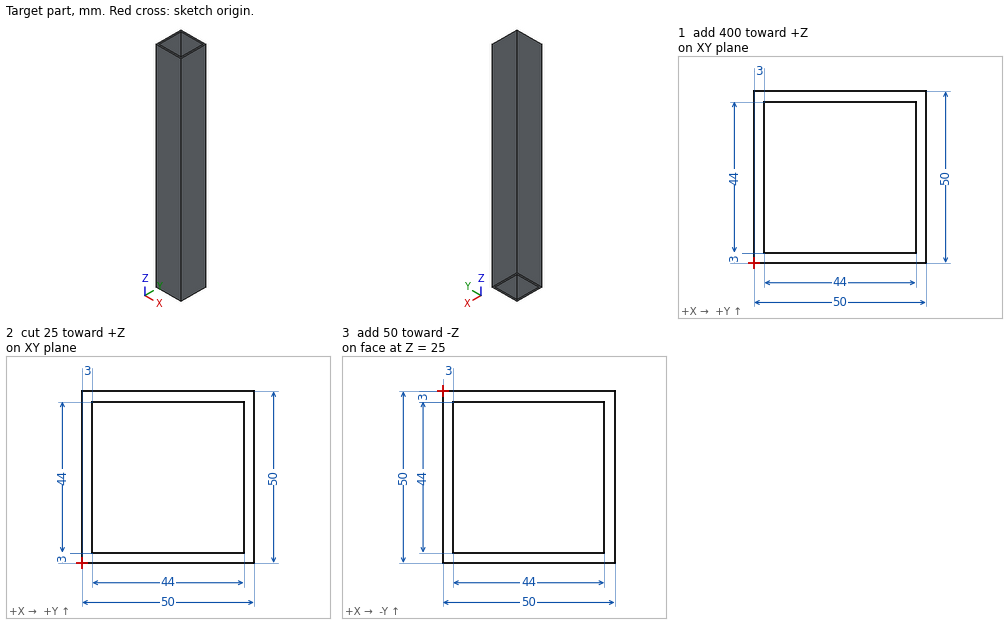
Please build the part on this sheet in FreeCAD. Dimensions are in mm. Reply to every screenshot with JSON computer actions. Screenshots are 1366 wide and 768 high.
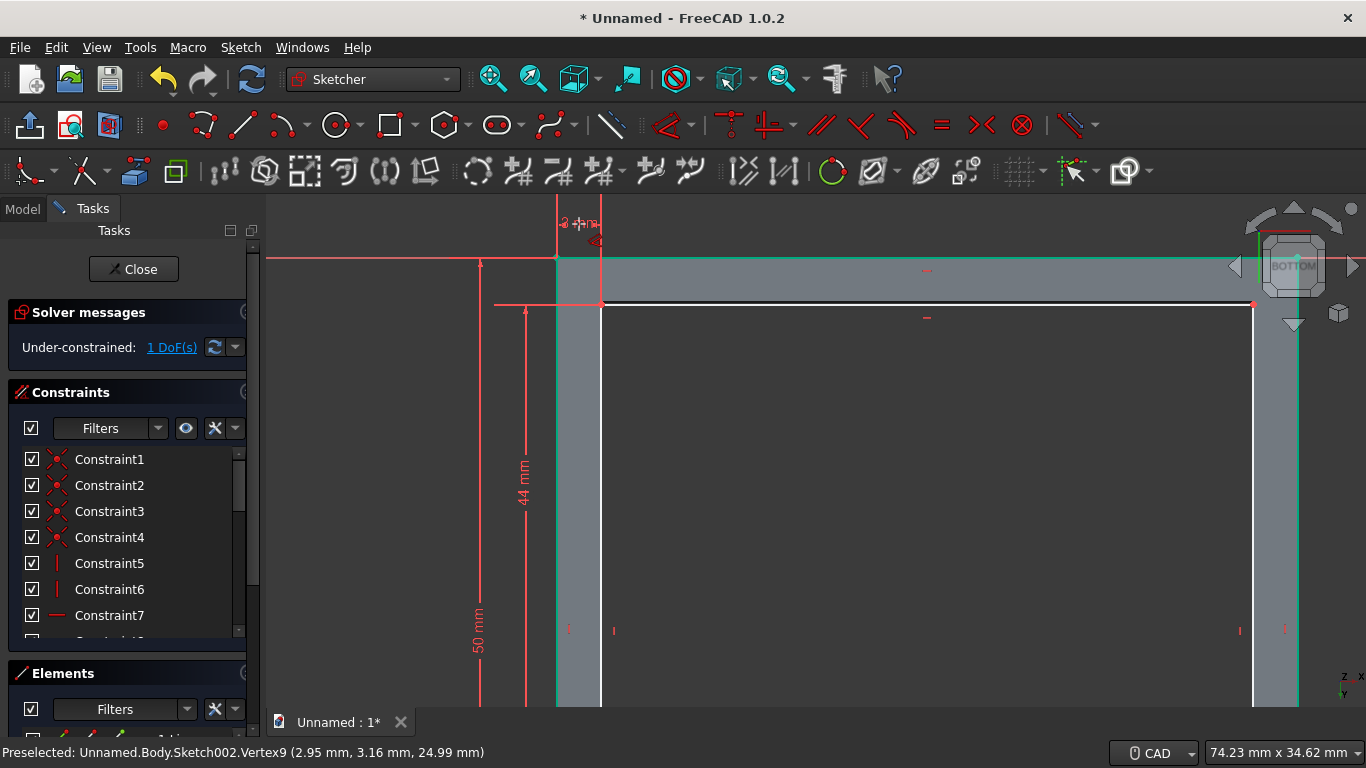
{"action": "left_click", "coordinate": [601, 305]}
{"action": "left_click", "coordinate": [523, 281]}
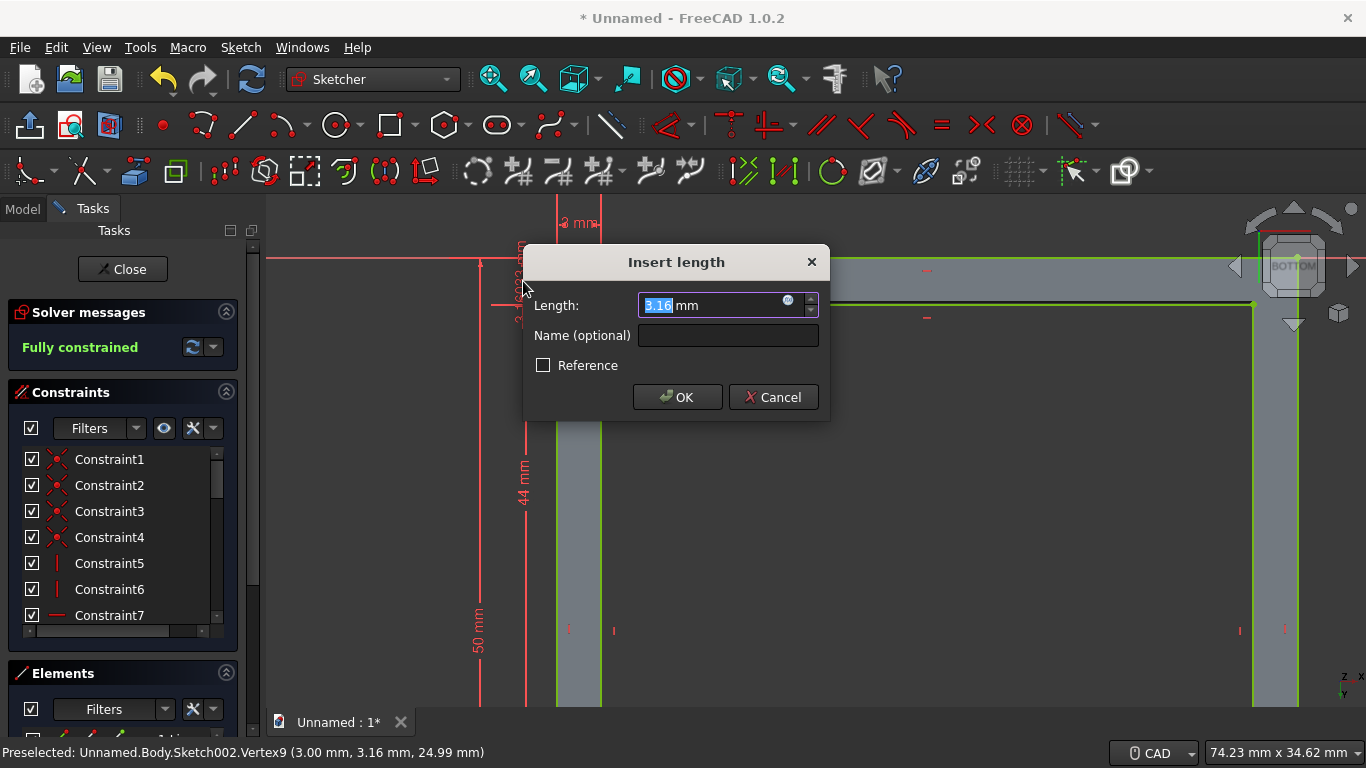
{"action": "type", "text": "3"}
{"action": "key", "text": "Return"}
{"action": "key", "text": "Escape"}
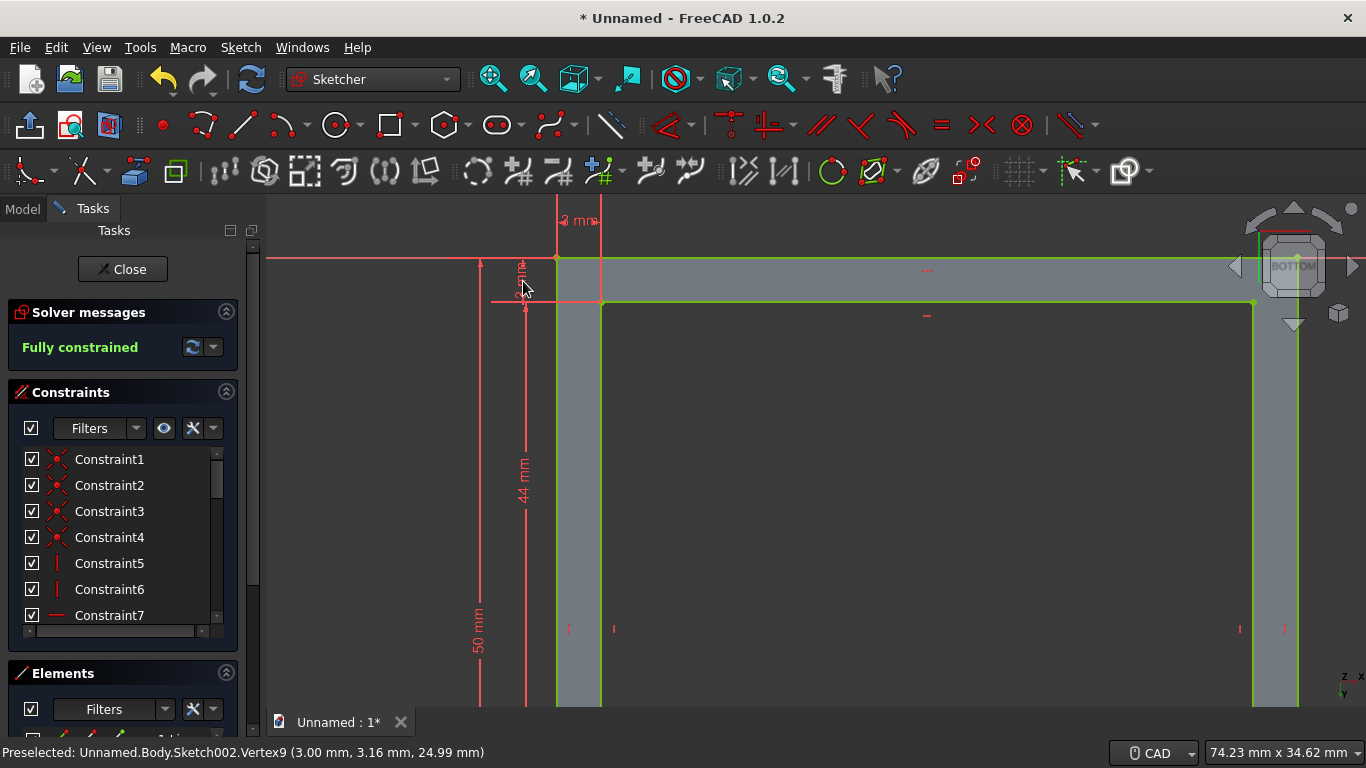
{"action": "left_click", "coordinate": [123, 269]}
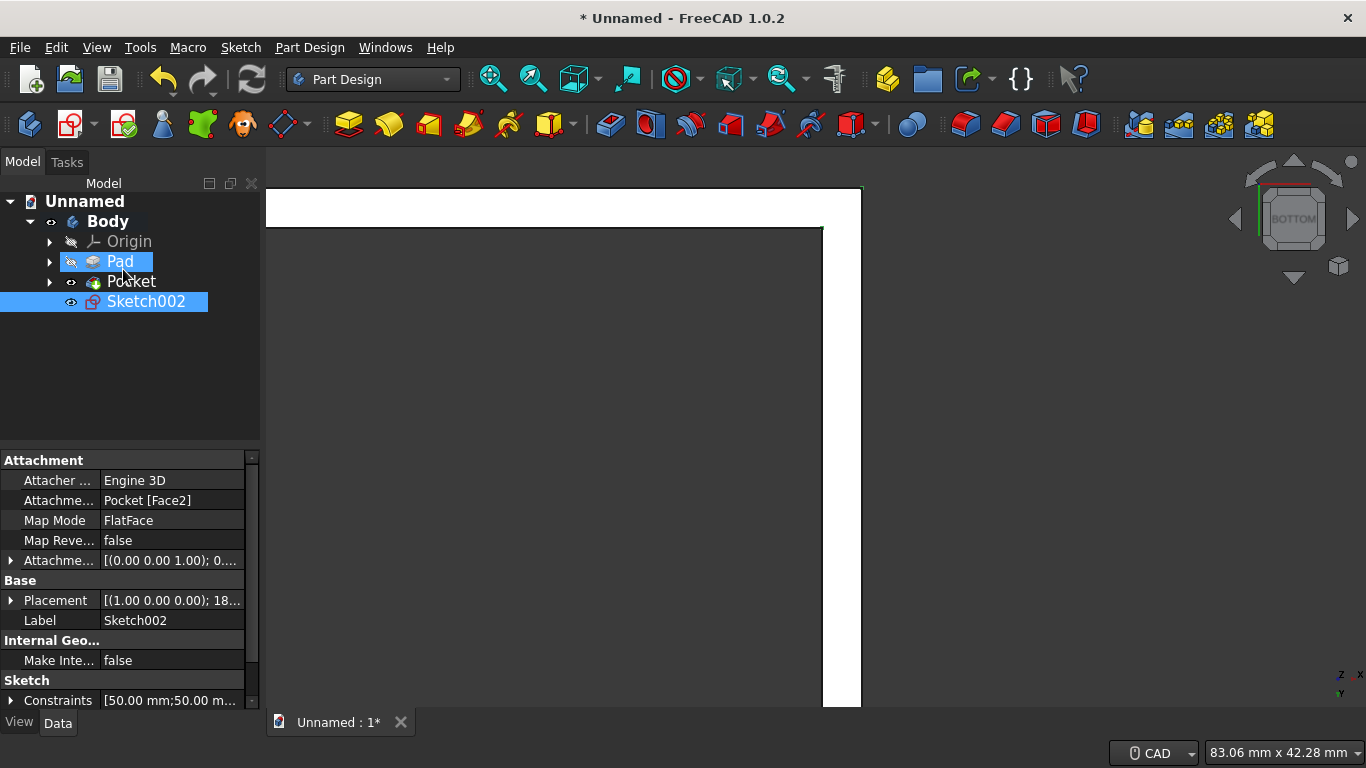
{"action": "left_click", "coordinate": [350, 124]}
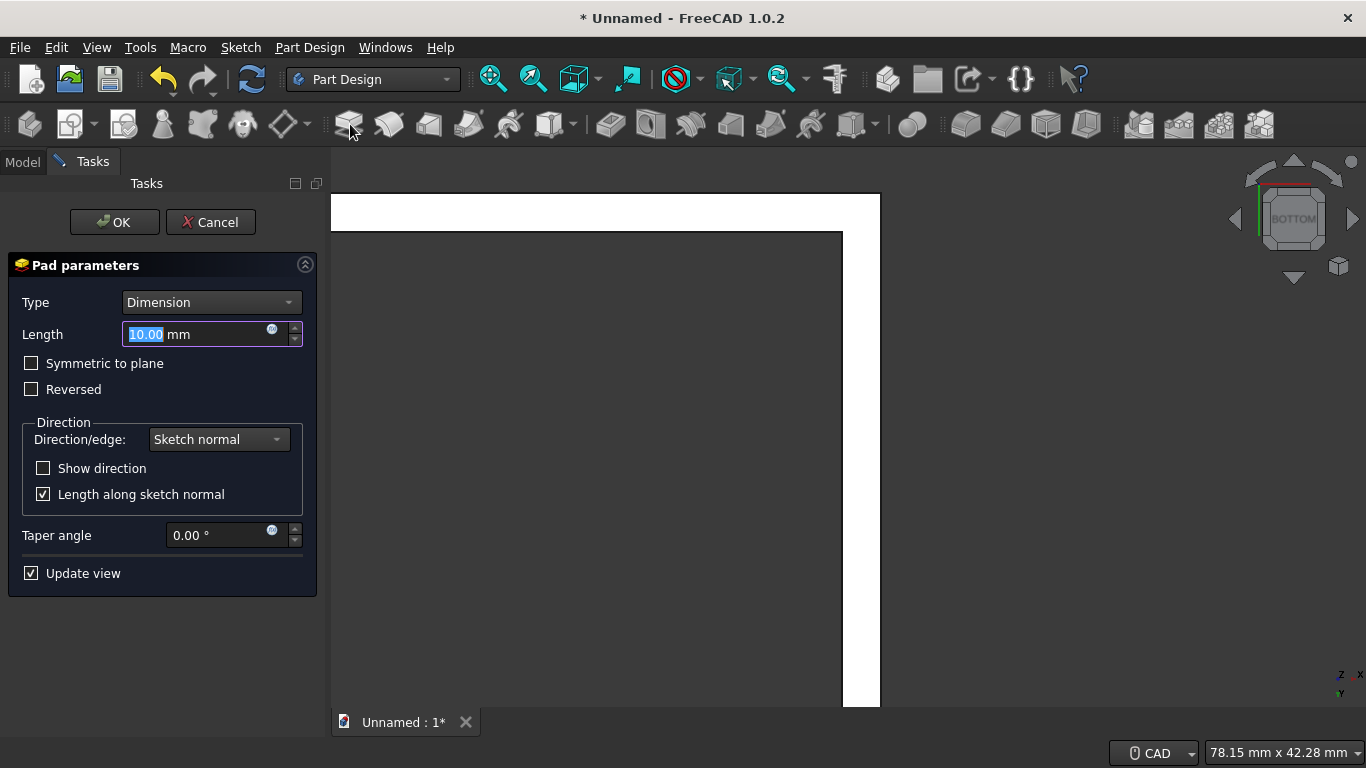
{"action": "type", "text": "50"}
{"action": "key", "text": "Tab"}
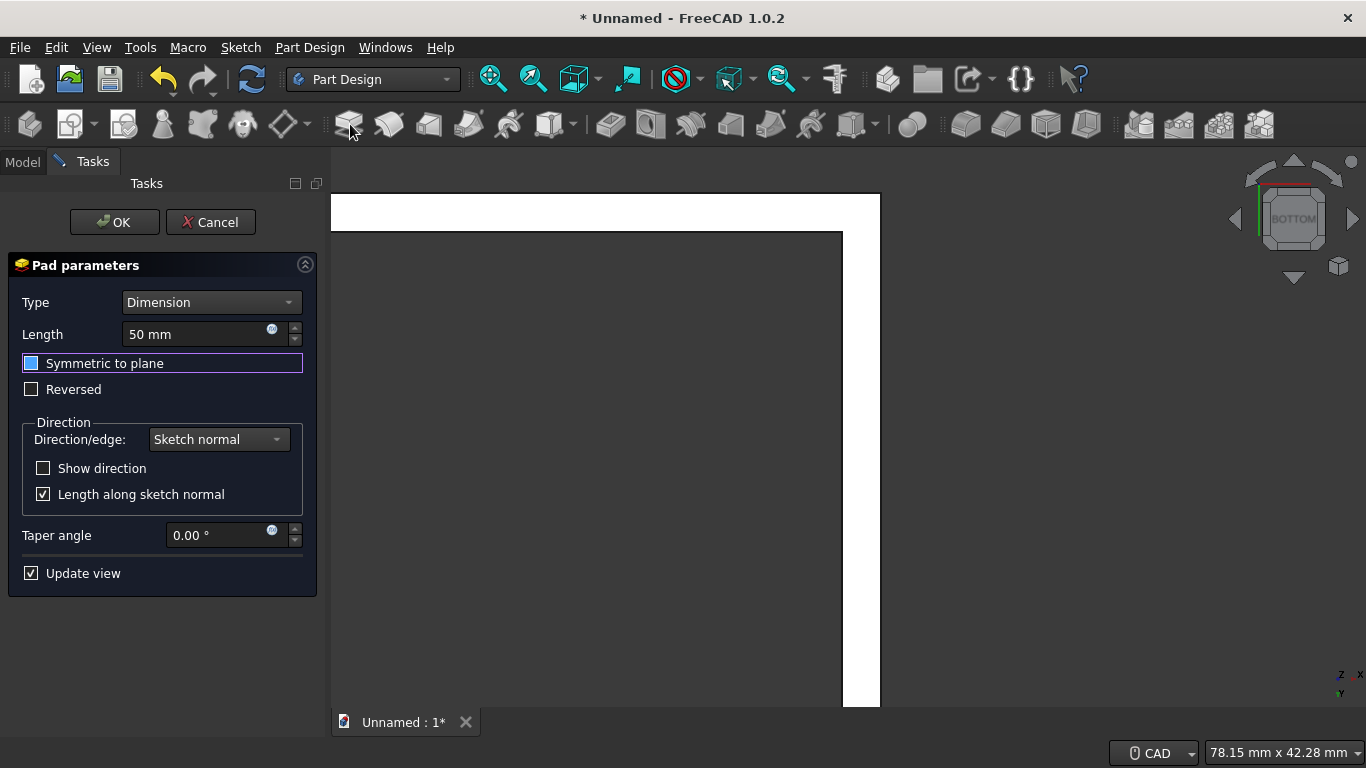
{"action": "left_click", "coordinate": [115, 222]}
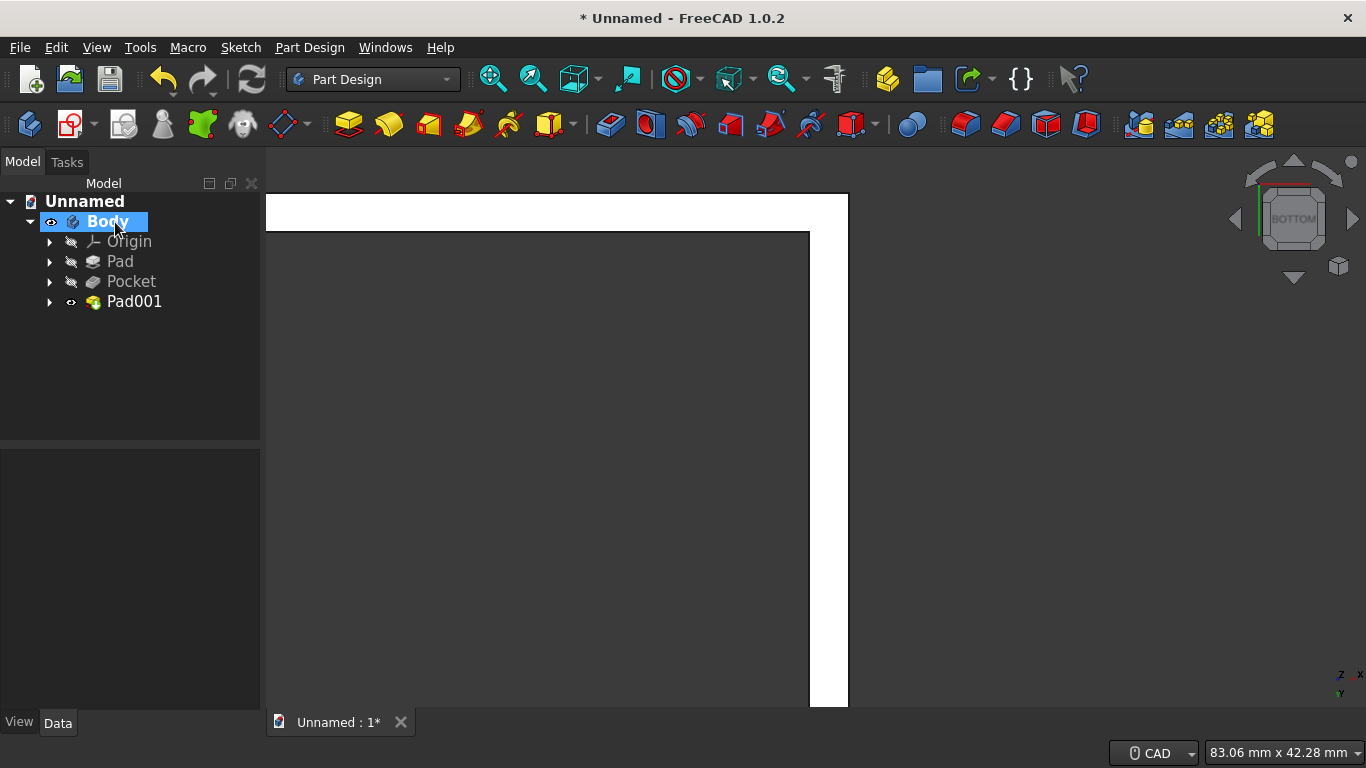
{"action": "key", "text": "0"}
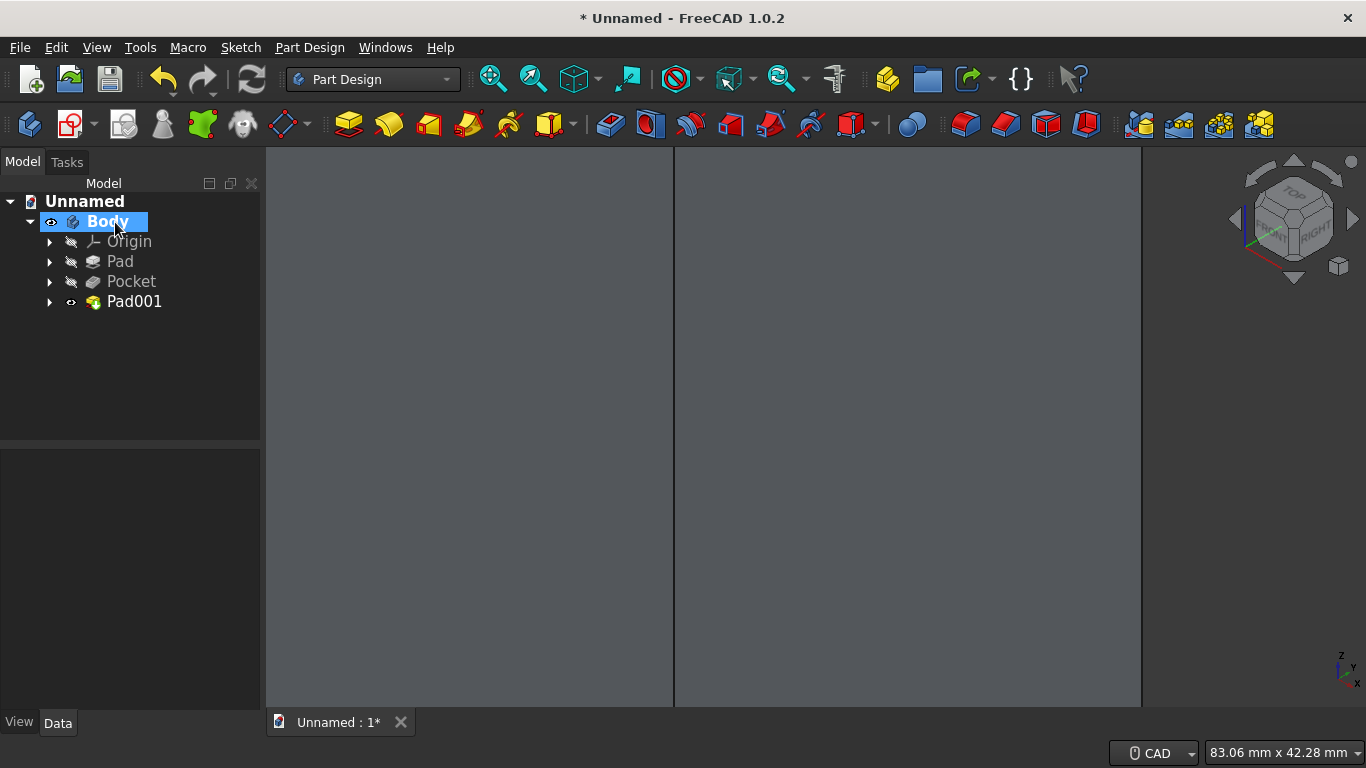
{"action": "left_click", "coordinate": [494, 80]}